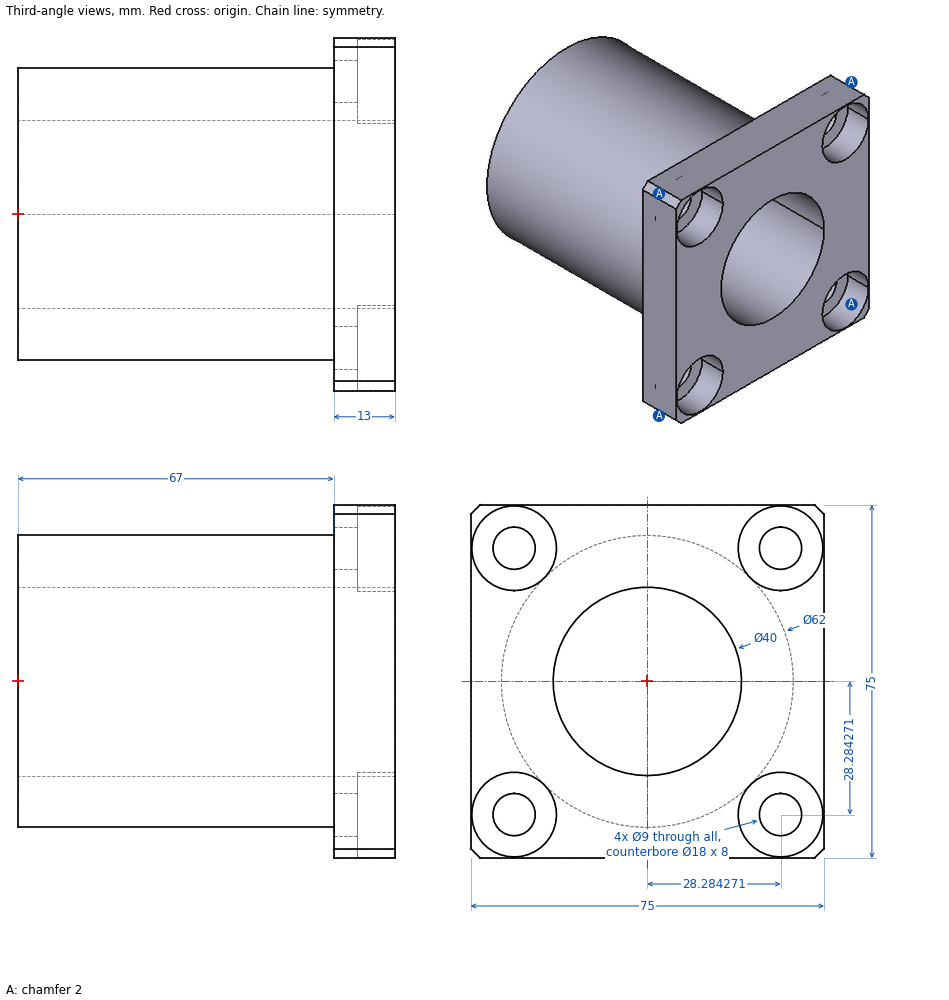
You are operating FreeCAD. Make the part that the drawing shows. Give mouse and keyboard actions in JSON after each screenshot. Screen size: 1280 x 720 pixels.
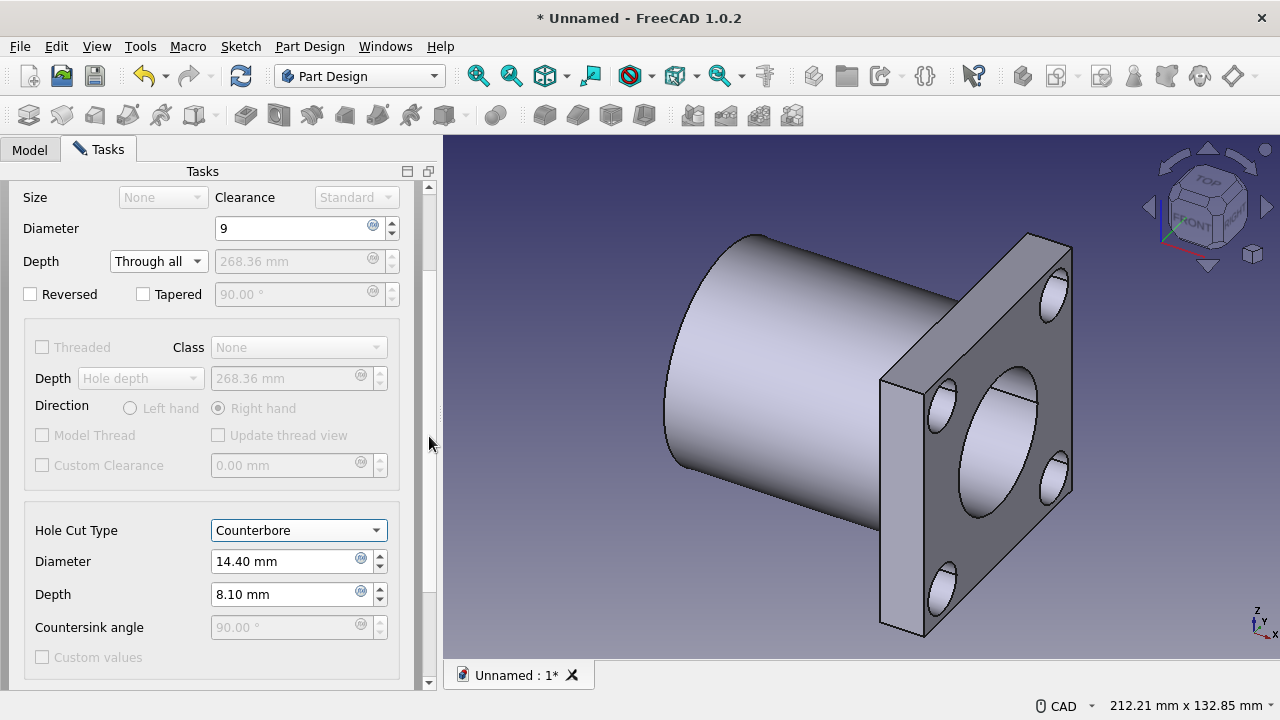
{"action": "triple_click", "coordinate": [292, 562]}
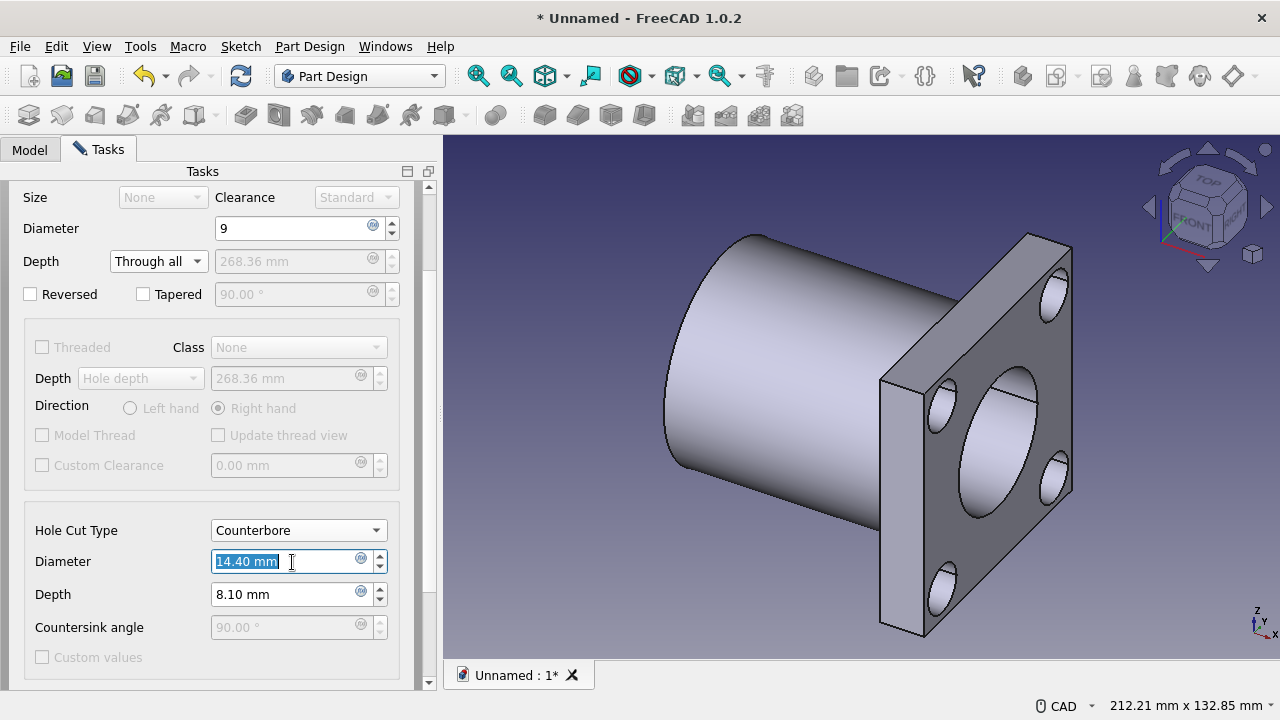
{"action": "type", "text": "18"}
{"action": "key", "text": "Tab"}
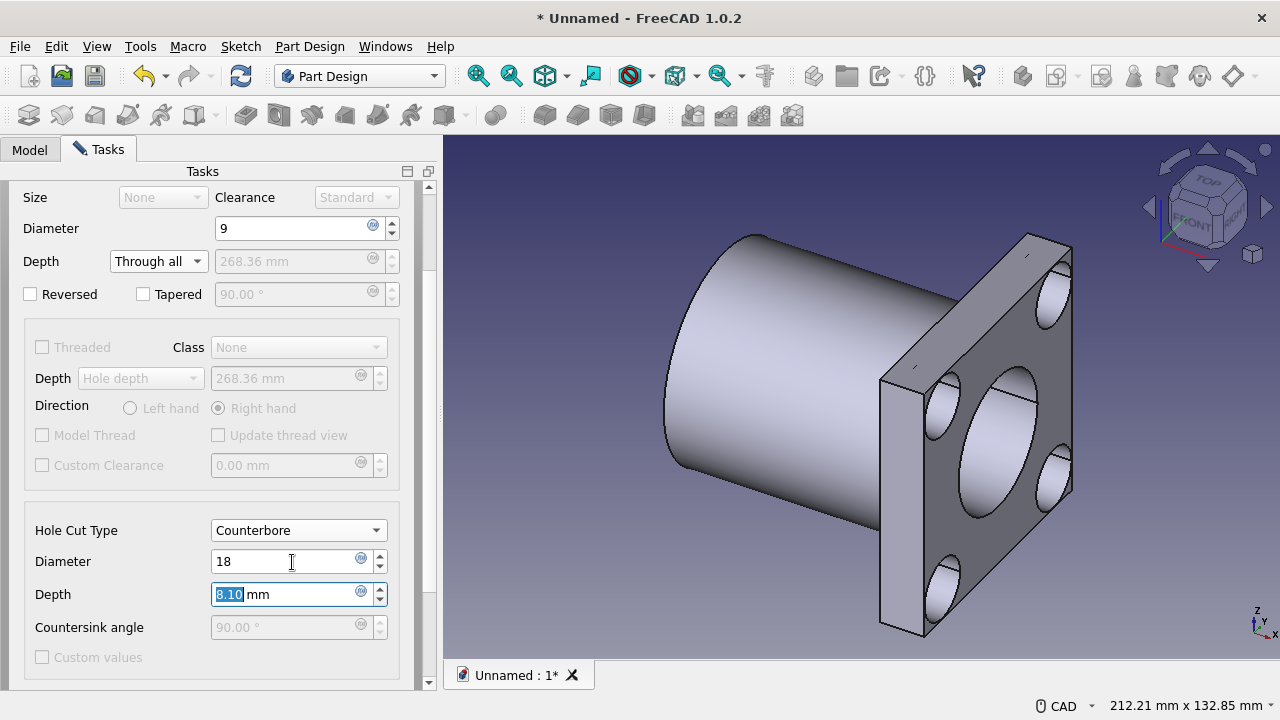
{"action": "type", "text": "8"}
{"action": "key", "text": "Tab"}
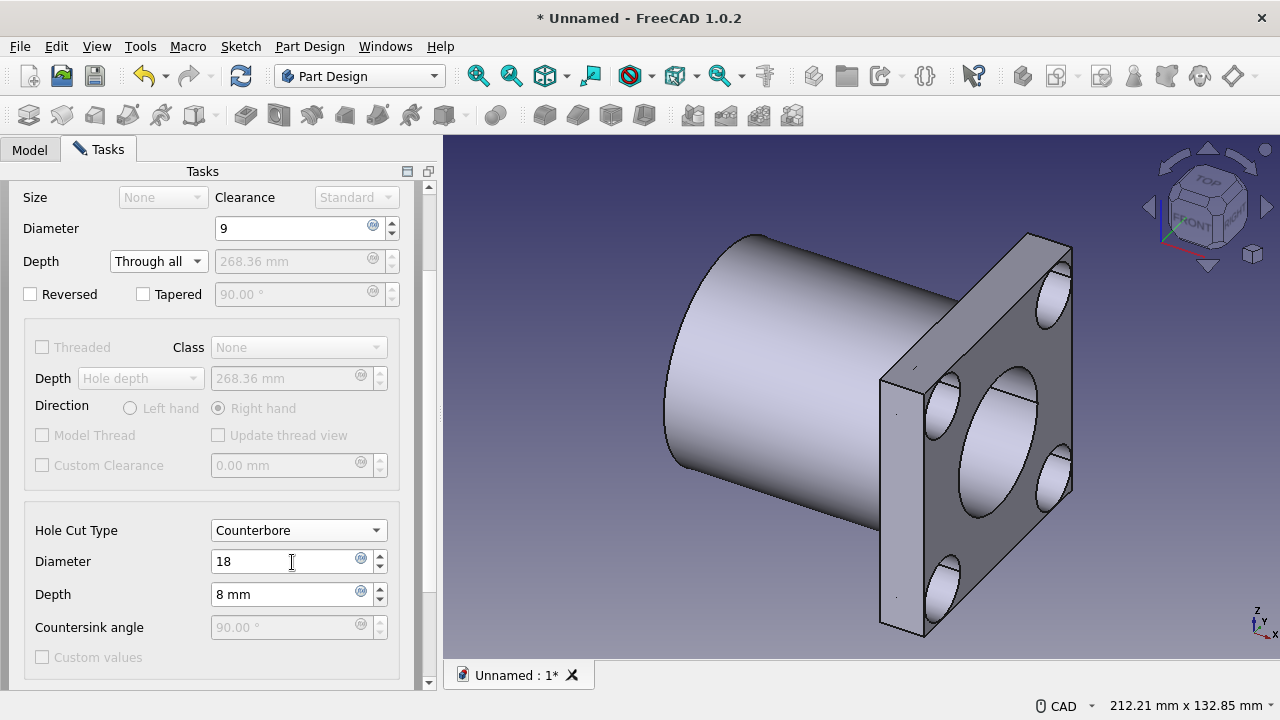
{"action": "scroll", "coordinate": [429, 436], "scroll_direction": "up", "scroll_amount": 3}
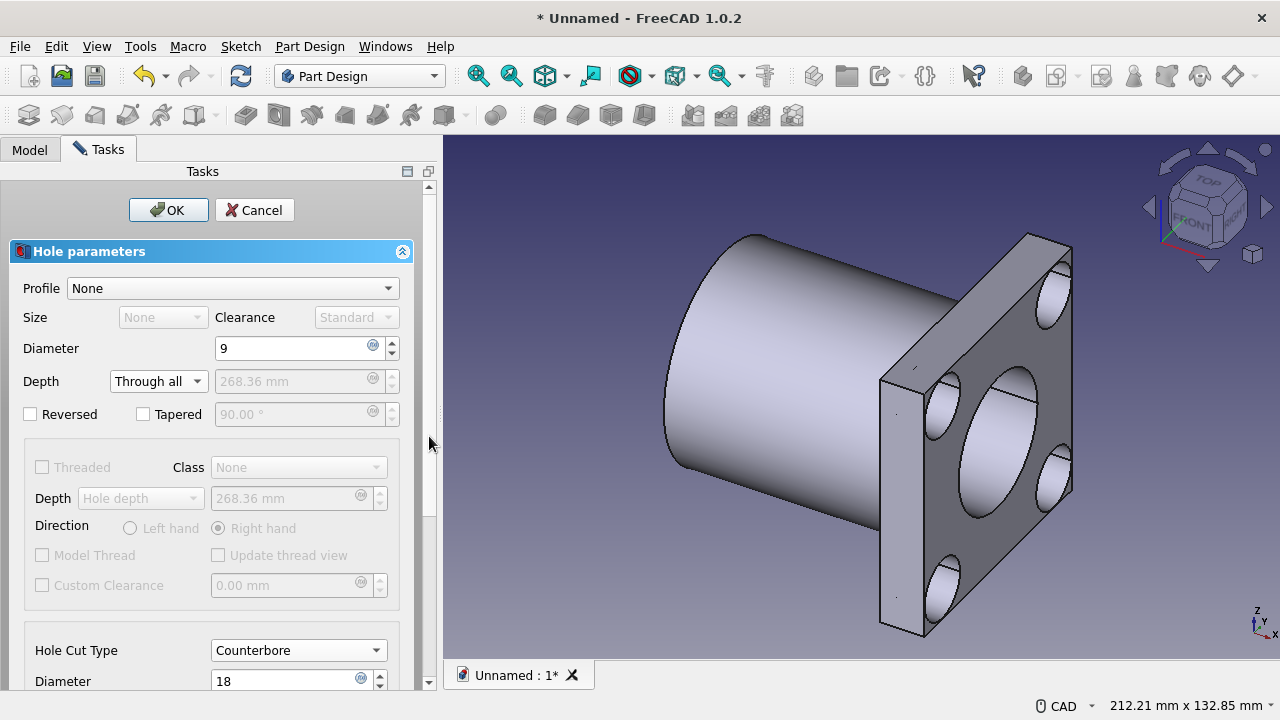
{"action": "left_click", "coordinate": [169, 210]}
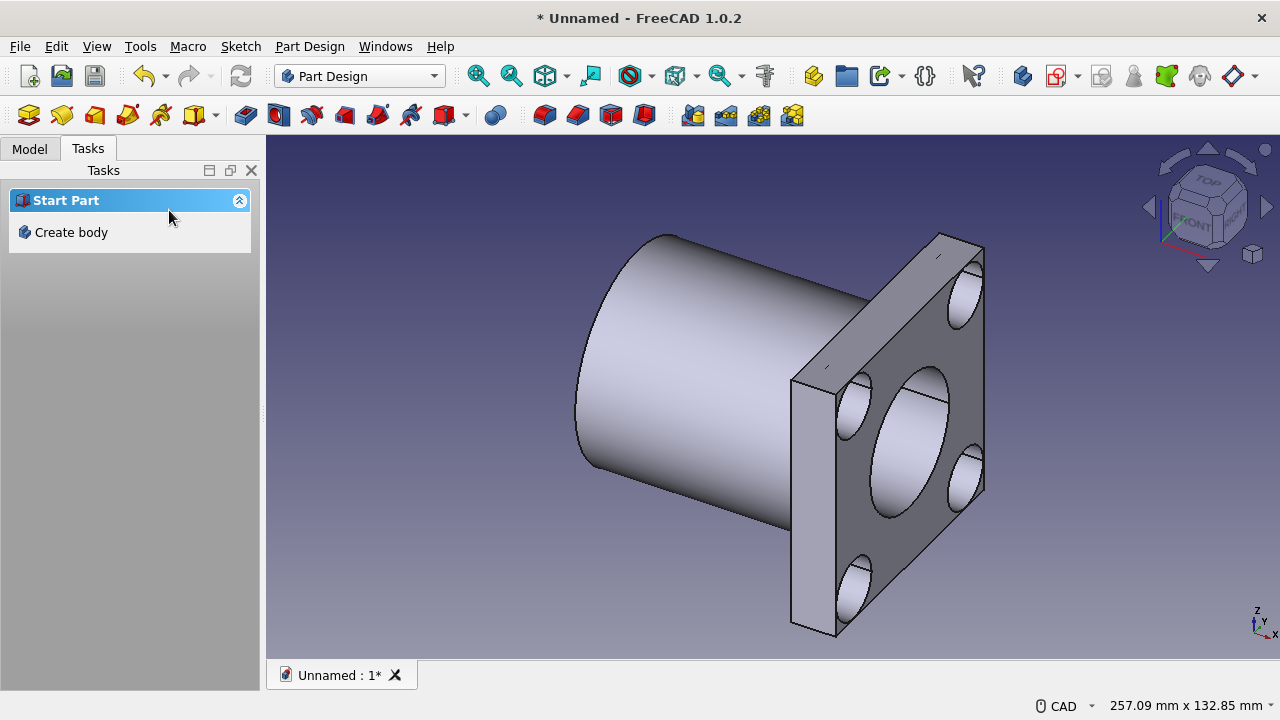
{"action": "left_click", "coordinate": [813, 386]}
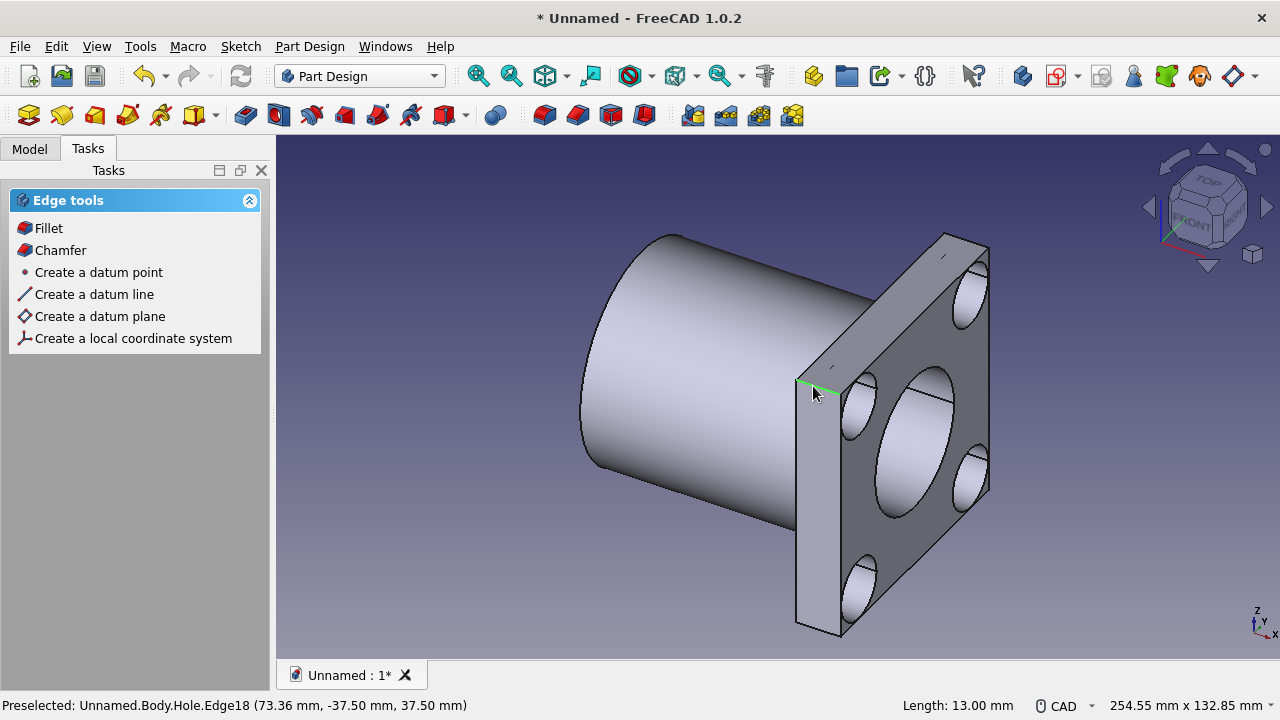
{"action": "key", "text": "0"}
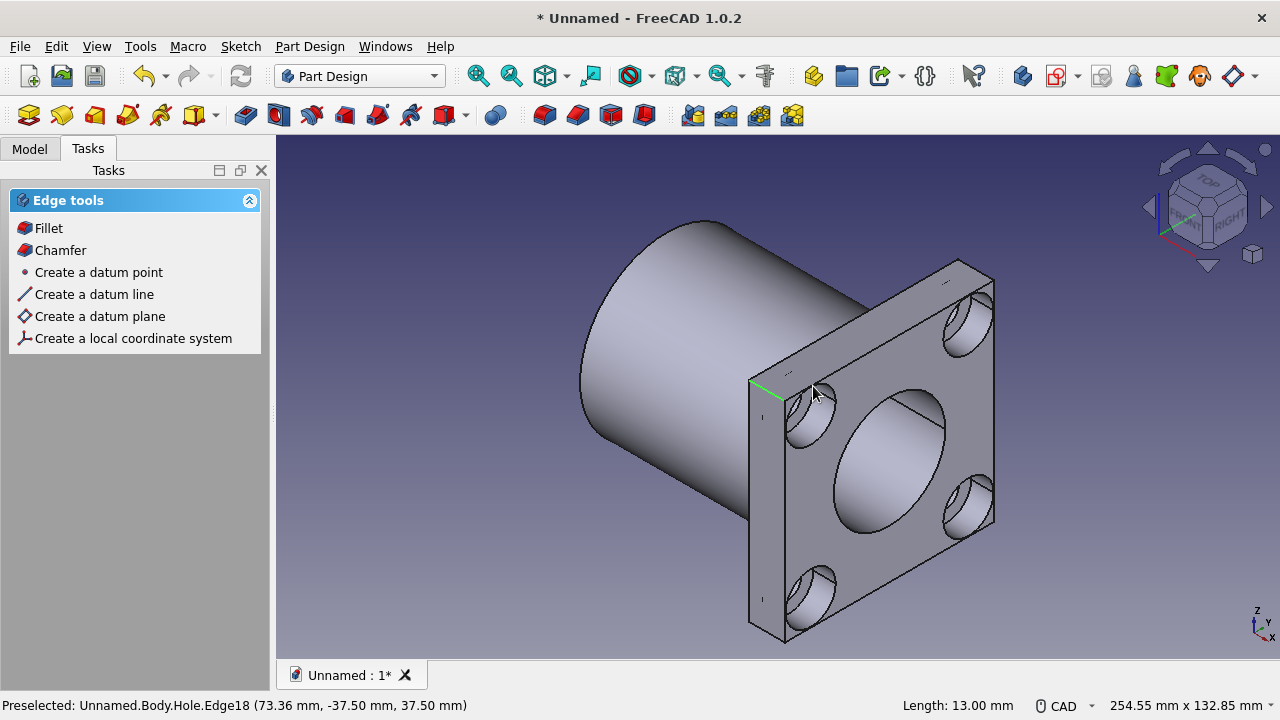
{"action": "key", "text": "2"}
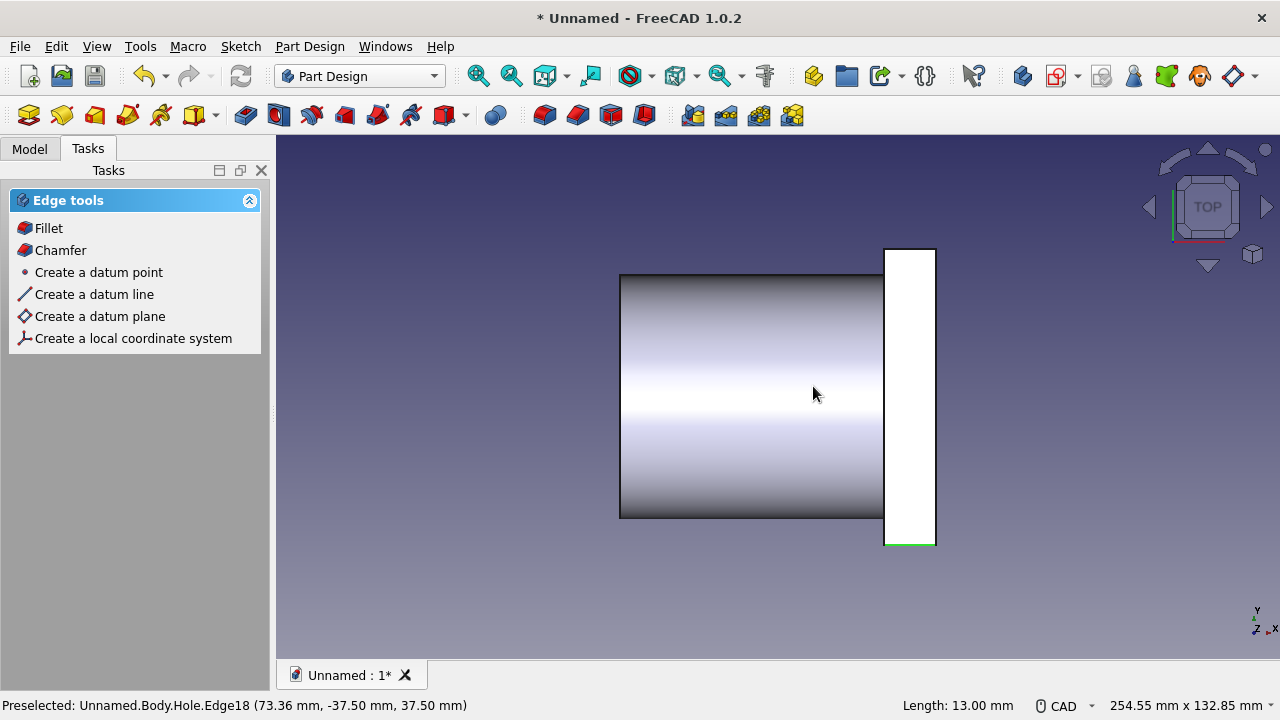
{"action": "left_click", "coordinate": [910, 248], "text": "ctrl"}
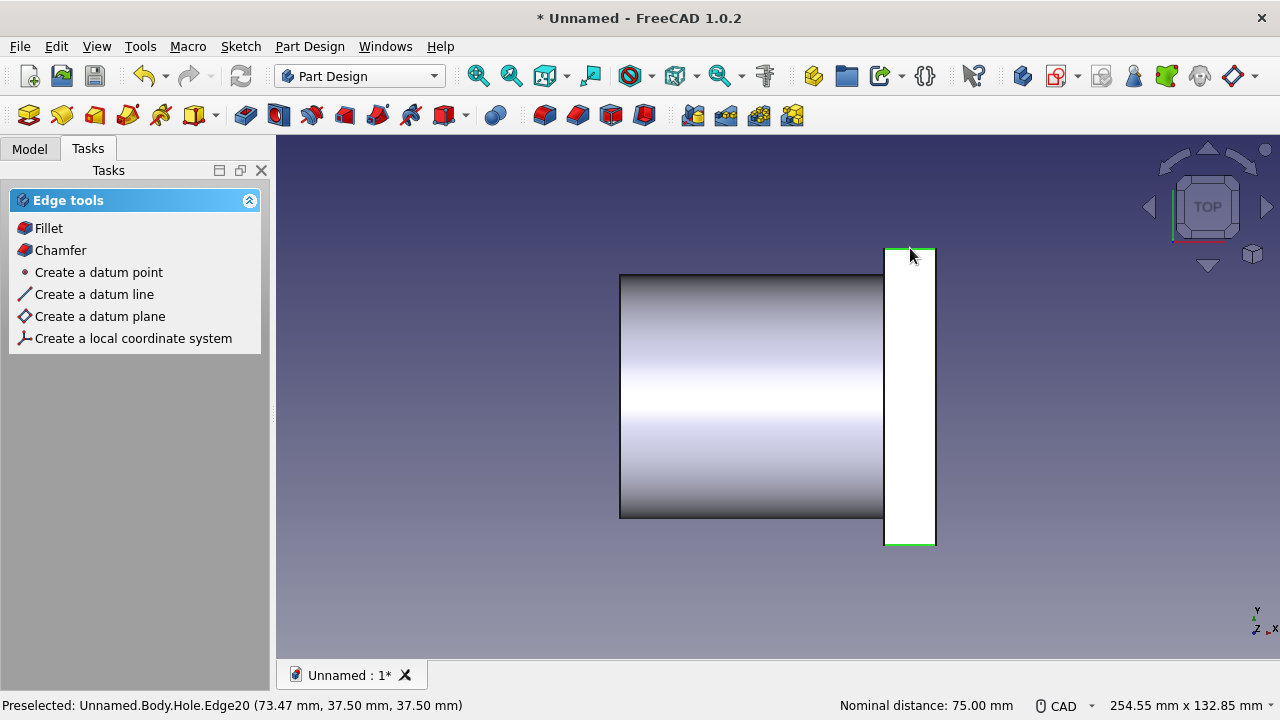
{"action": "key", "text": "1"}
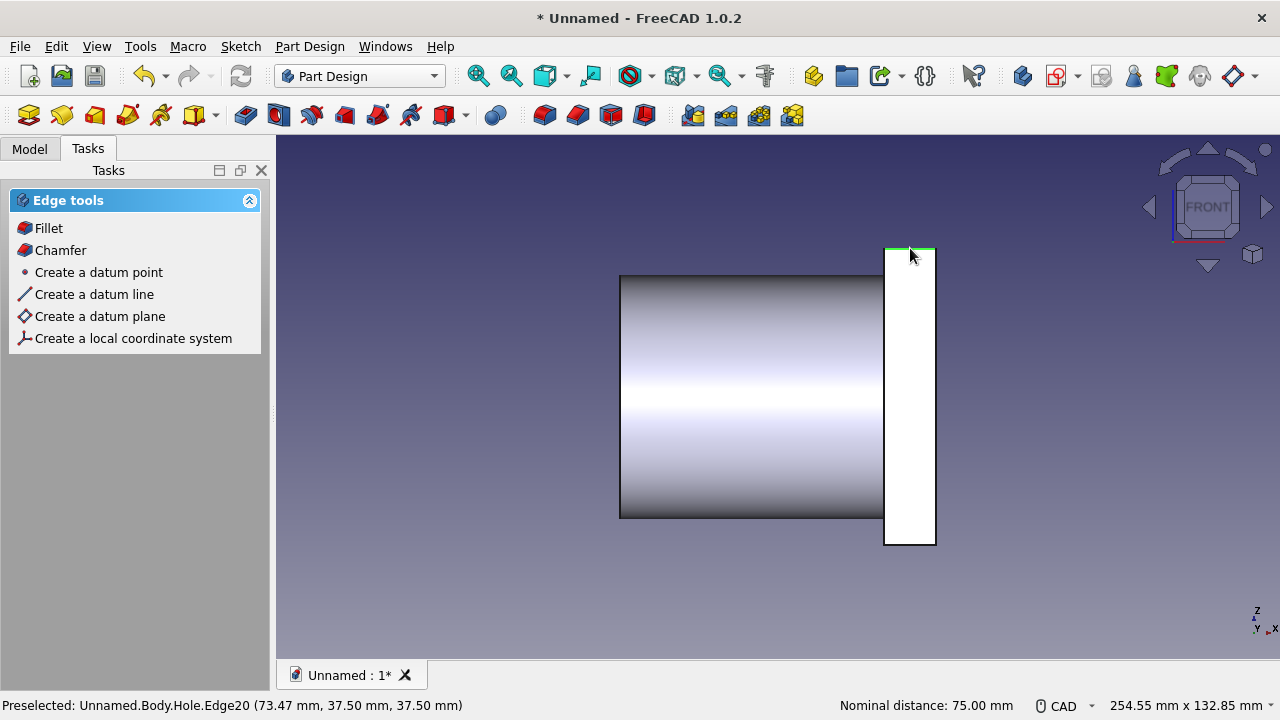
{"action": "left_click", "coordinate": [910, 544], "text": "ctrl"}